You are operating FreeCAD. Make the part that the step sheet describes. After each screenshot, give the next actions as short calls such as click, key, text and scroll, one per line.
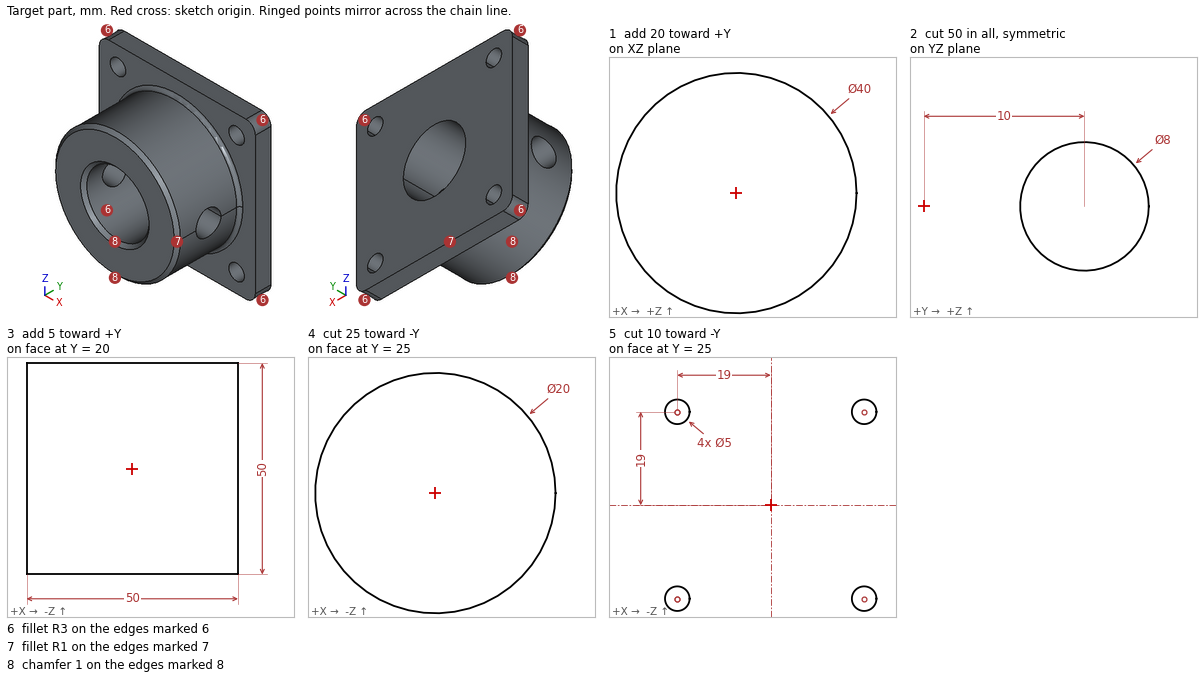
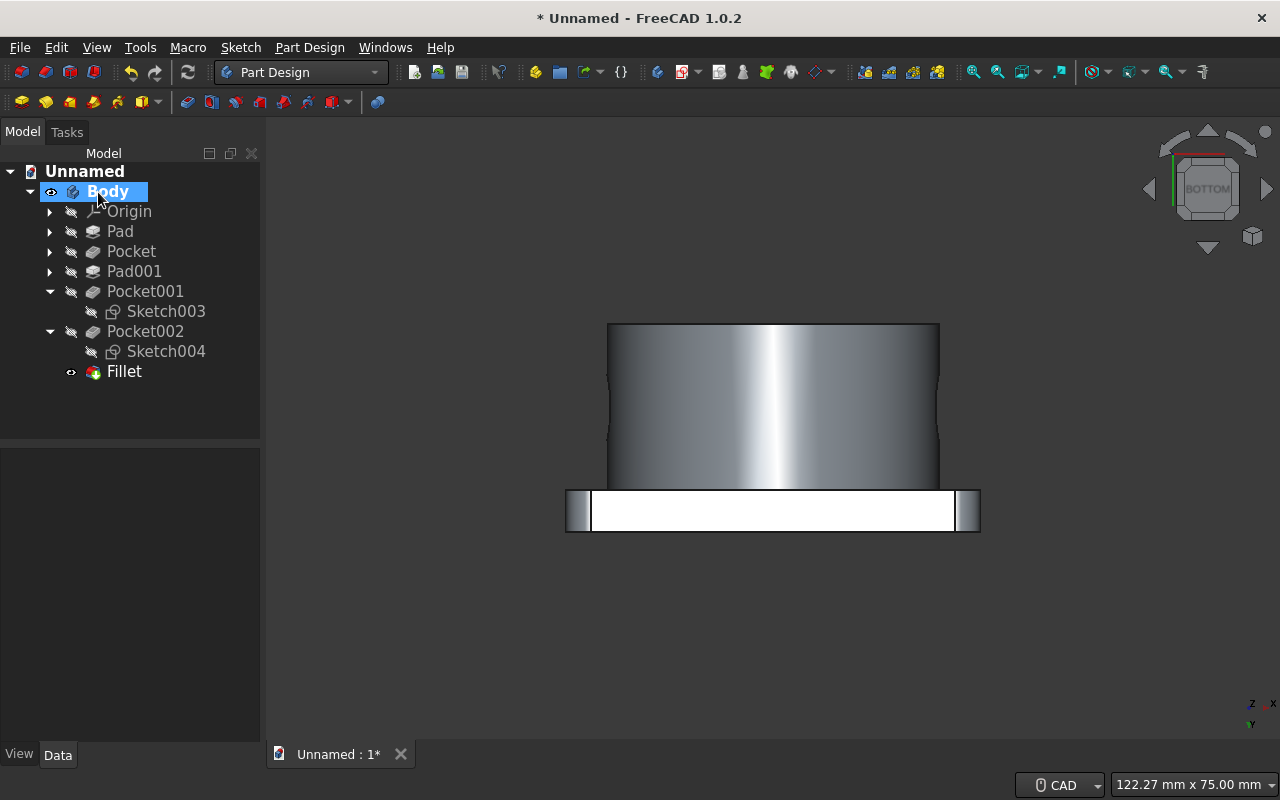
key(0)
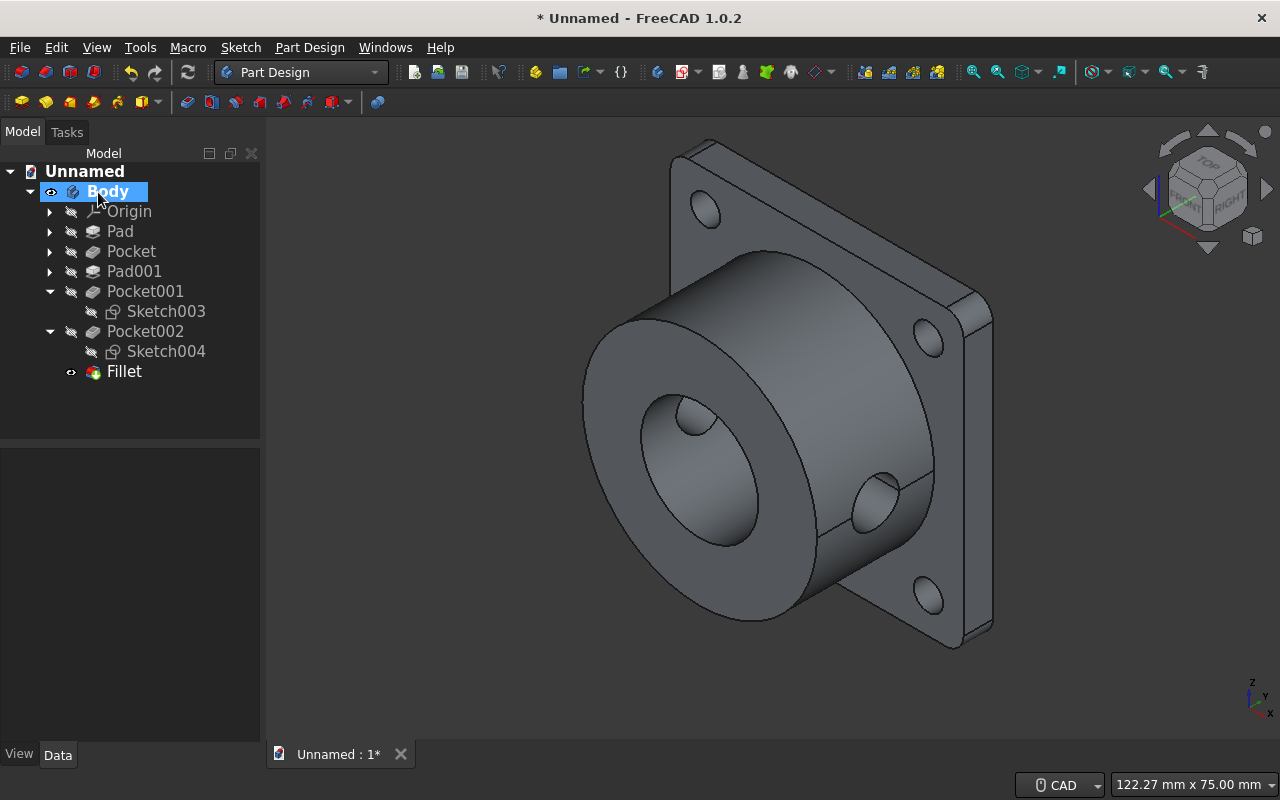
key(2)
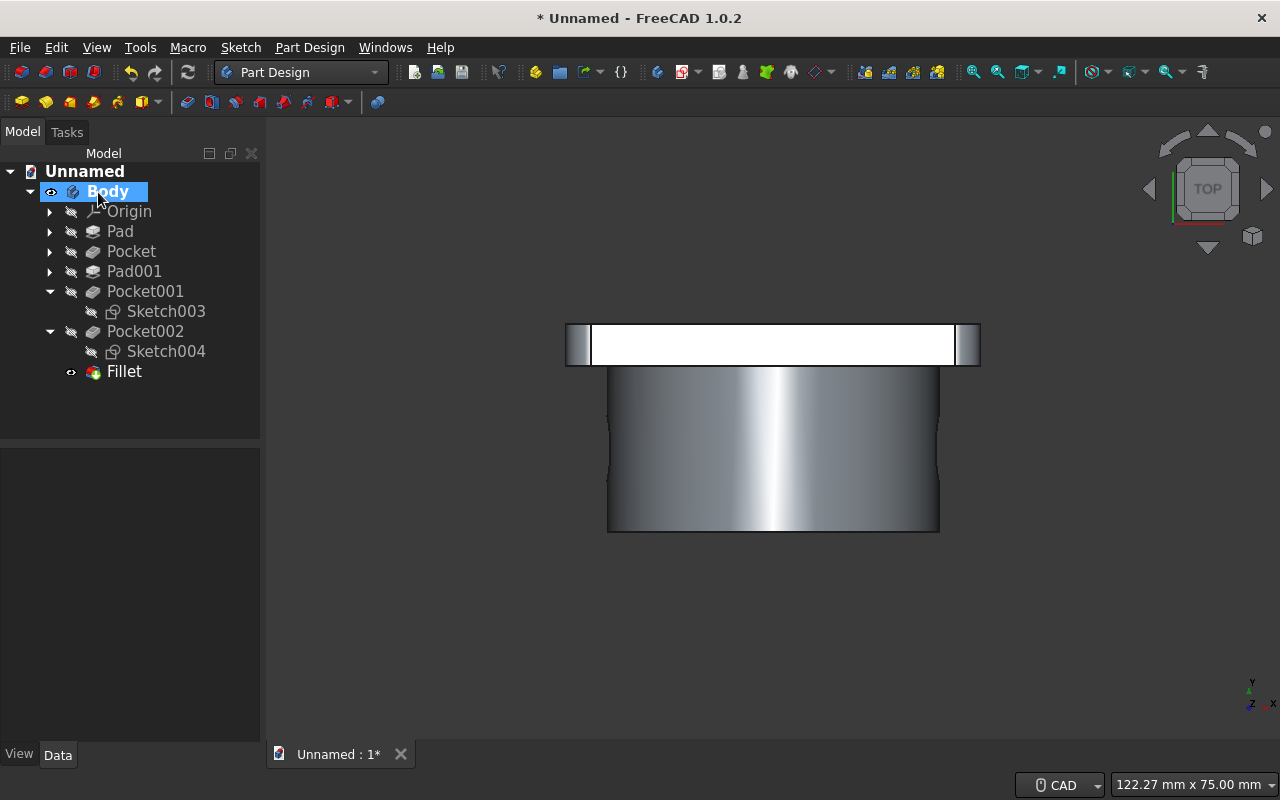
key(v)
key(f)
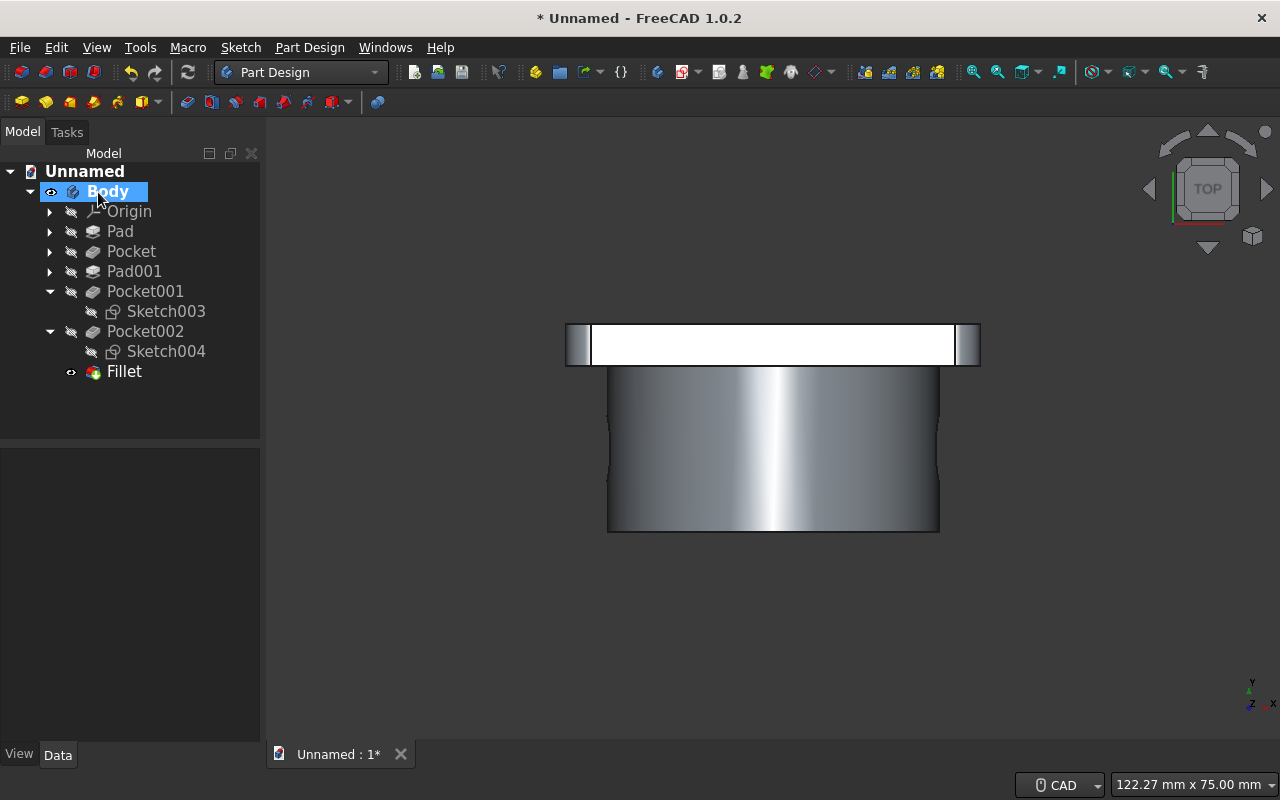
key(1)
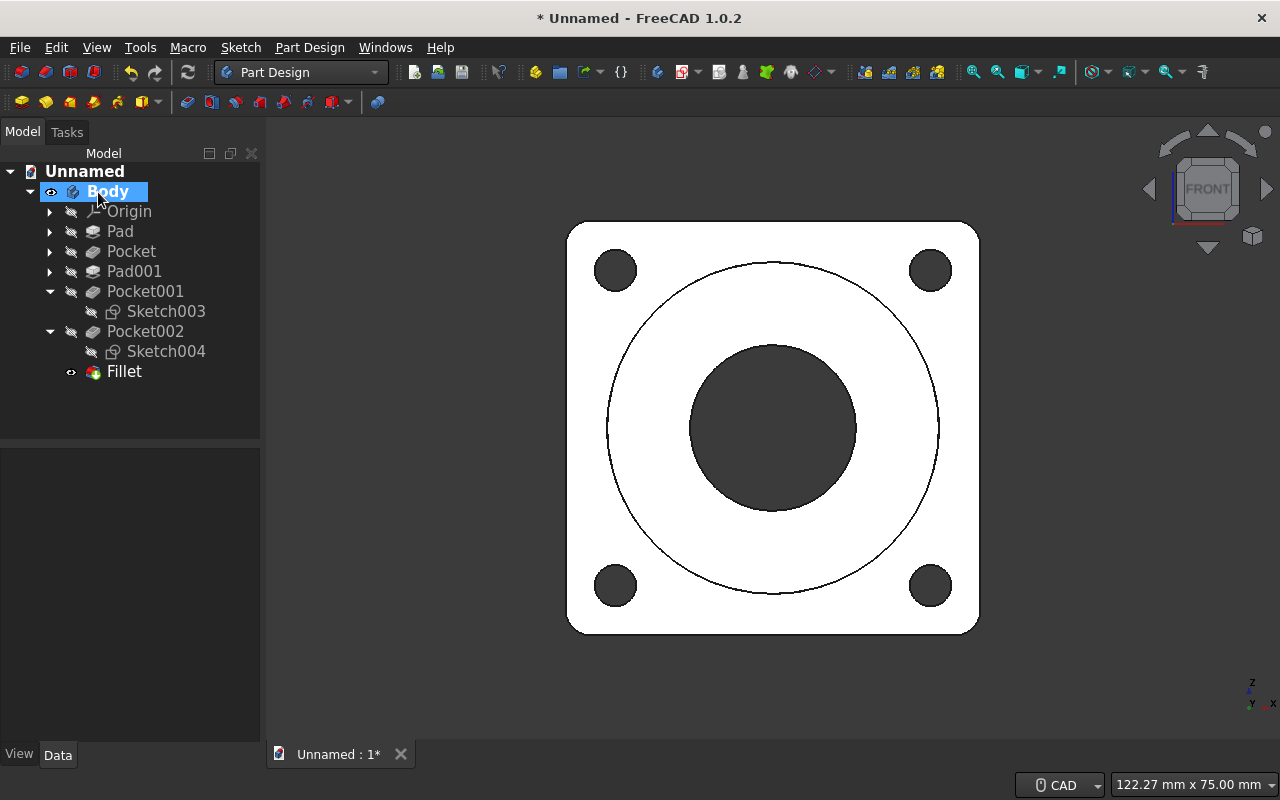
key(3)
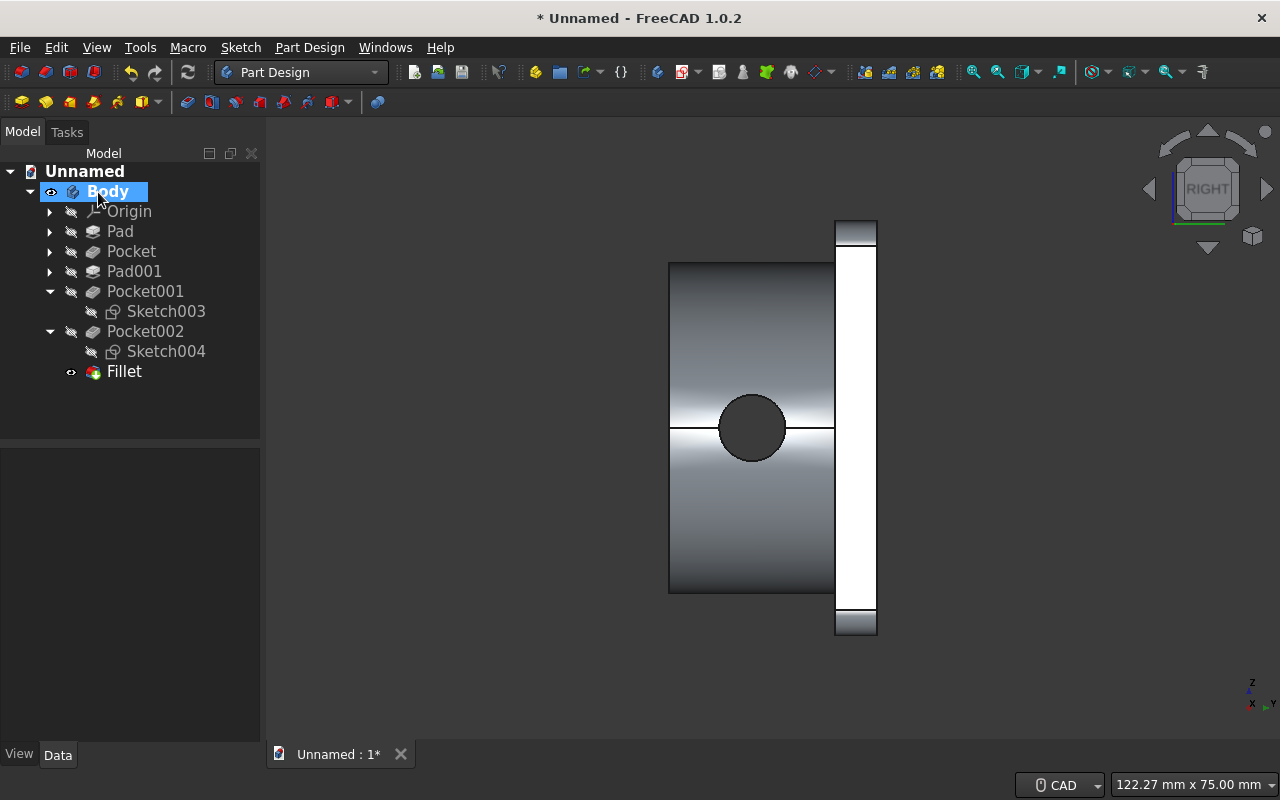
key(5)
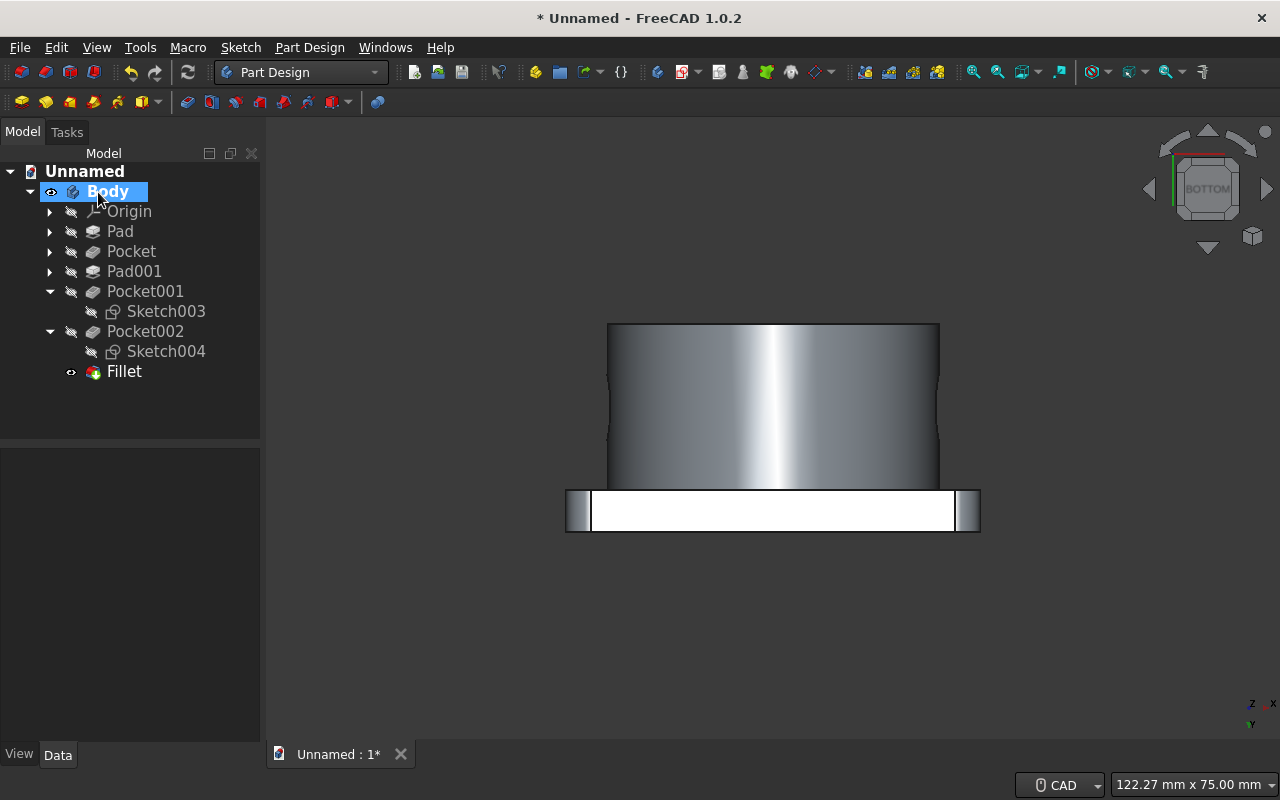
key(v)
key(f)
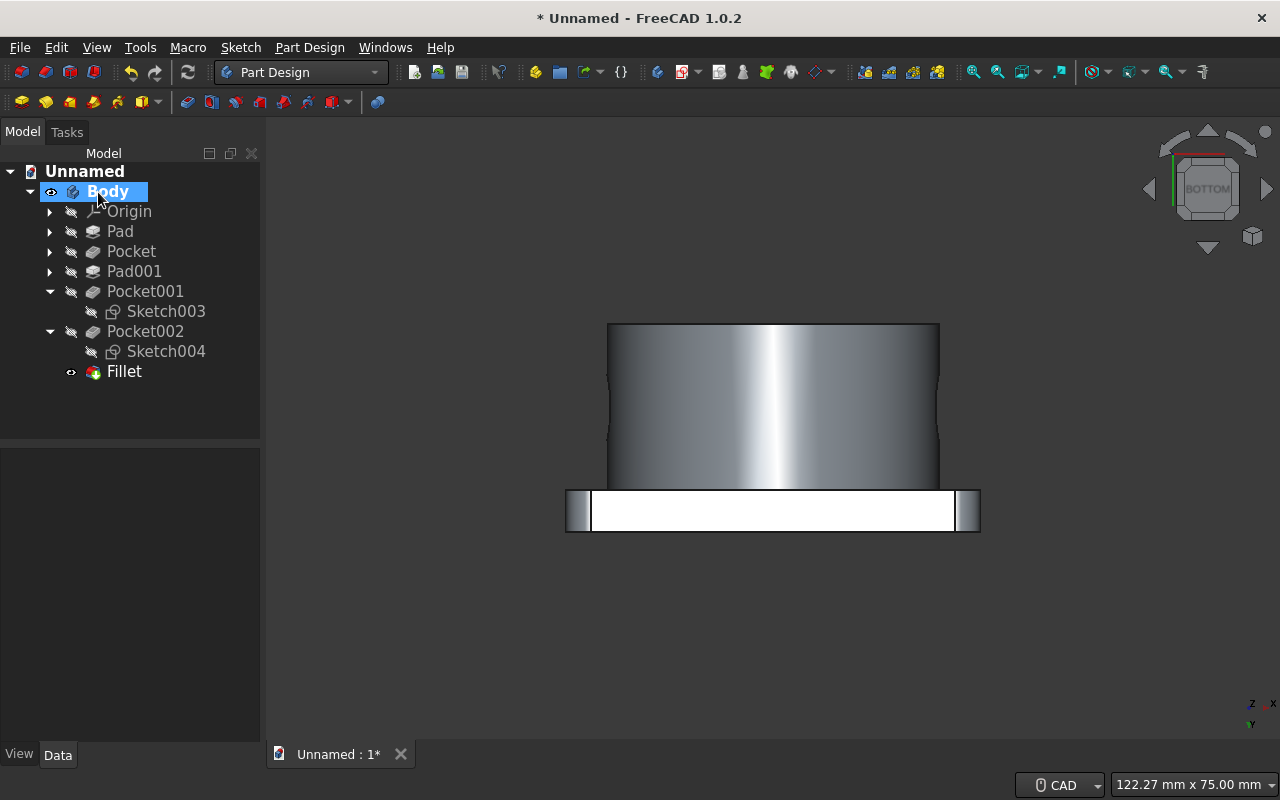
key(4)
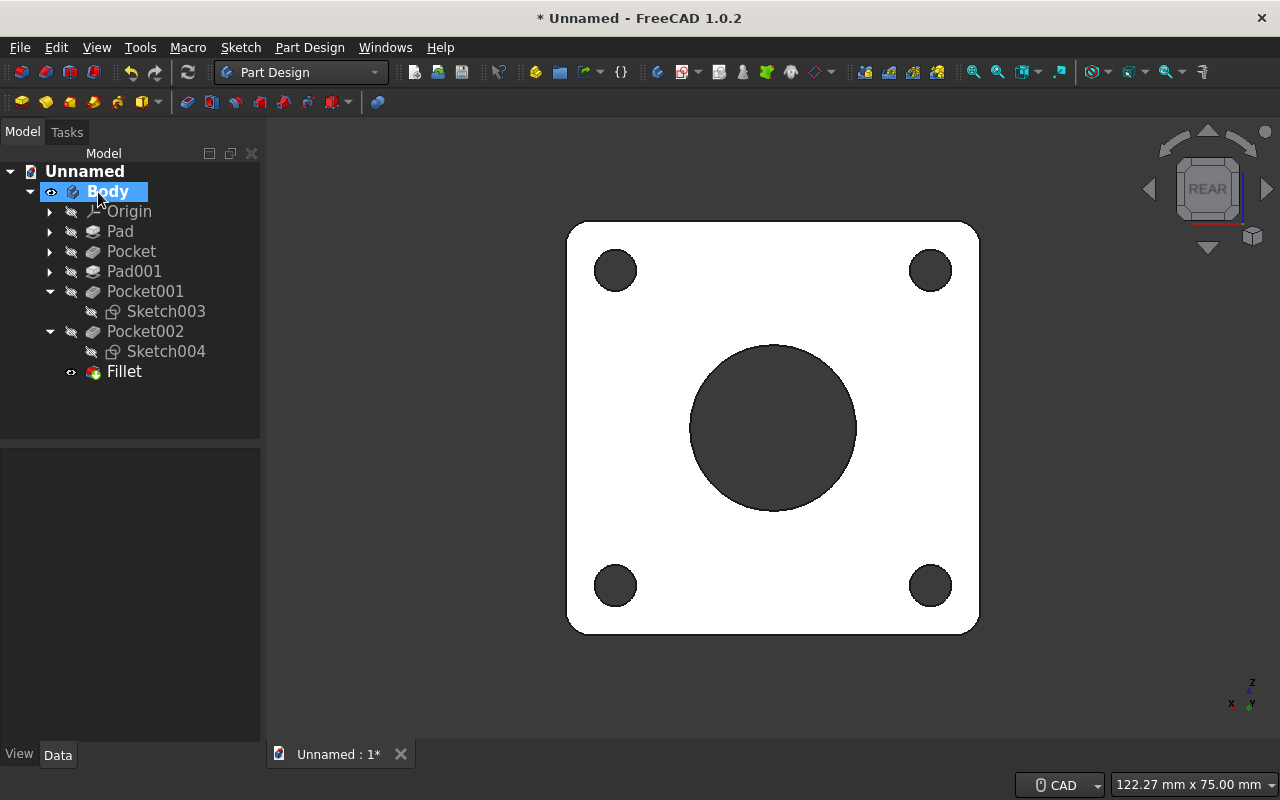
key(6)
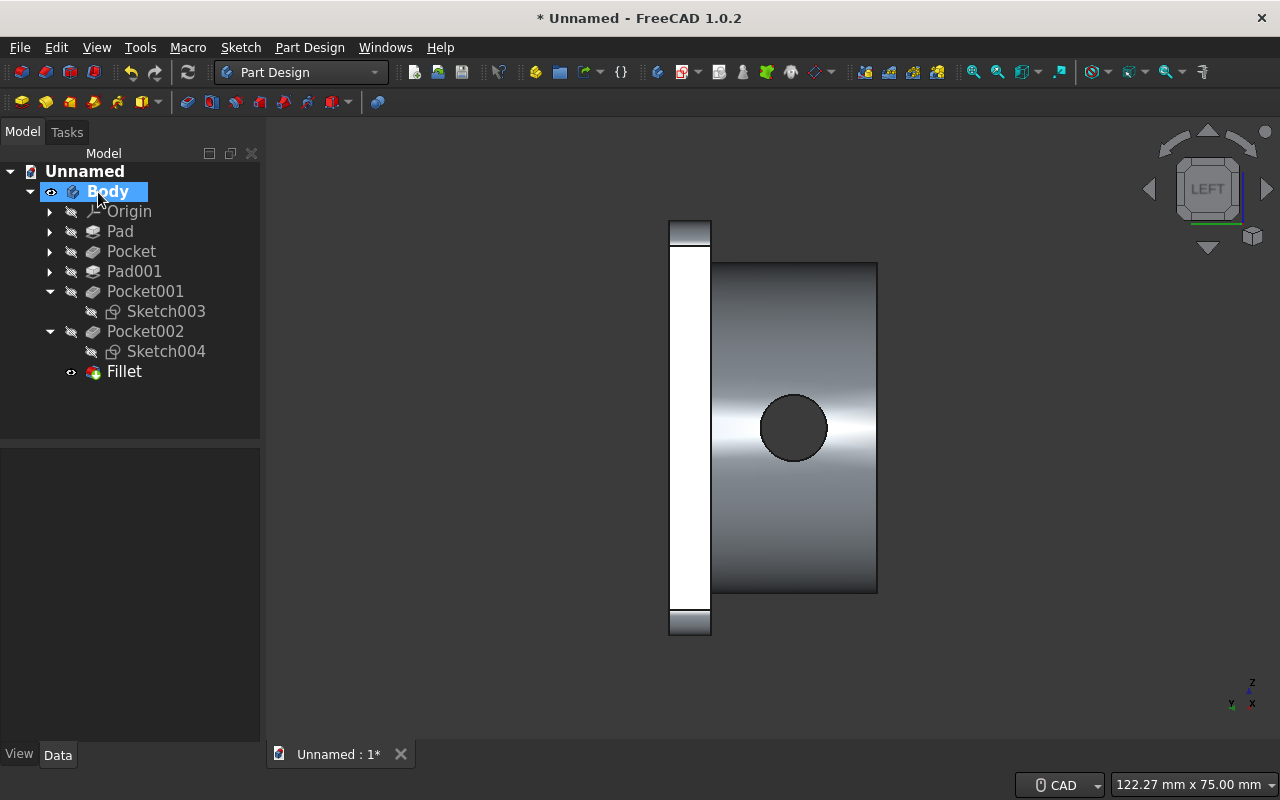
key(v)
key(3)